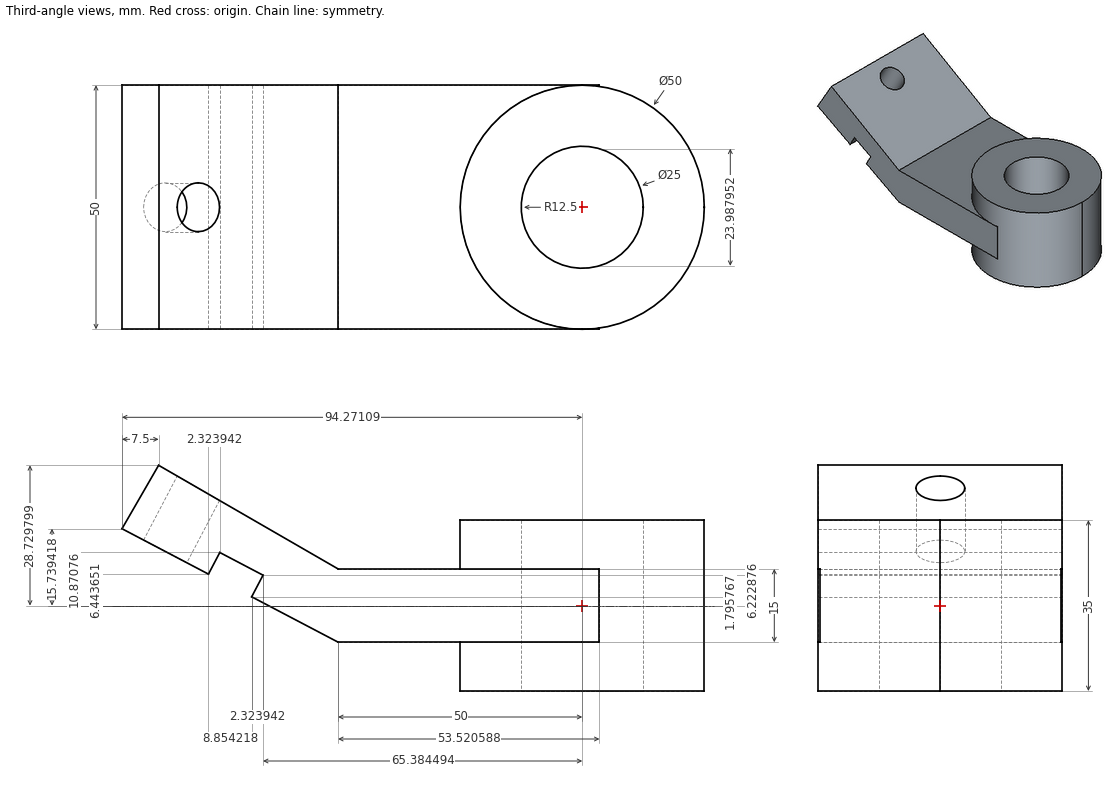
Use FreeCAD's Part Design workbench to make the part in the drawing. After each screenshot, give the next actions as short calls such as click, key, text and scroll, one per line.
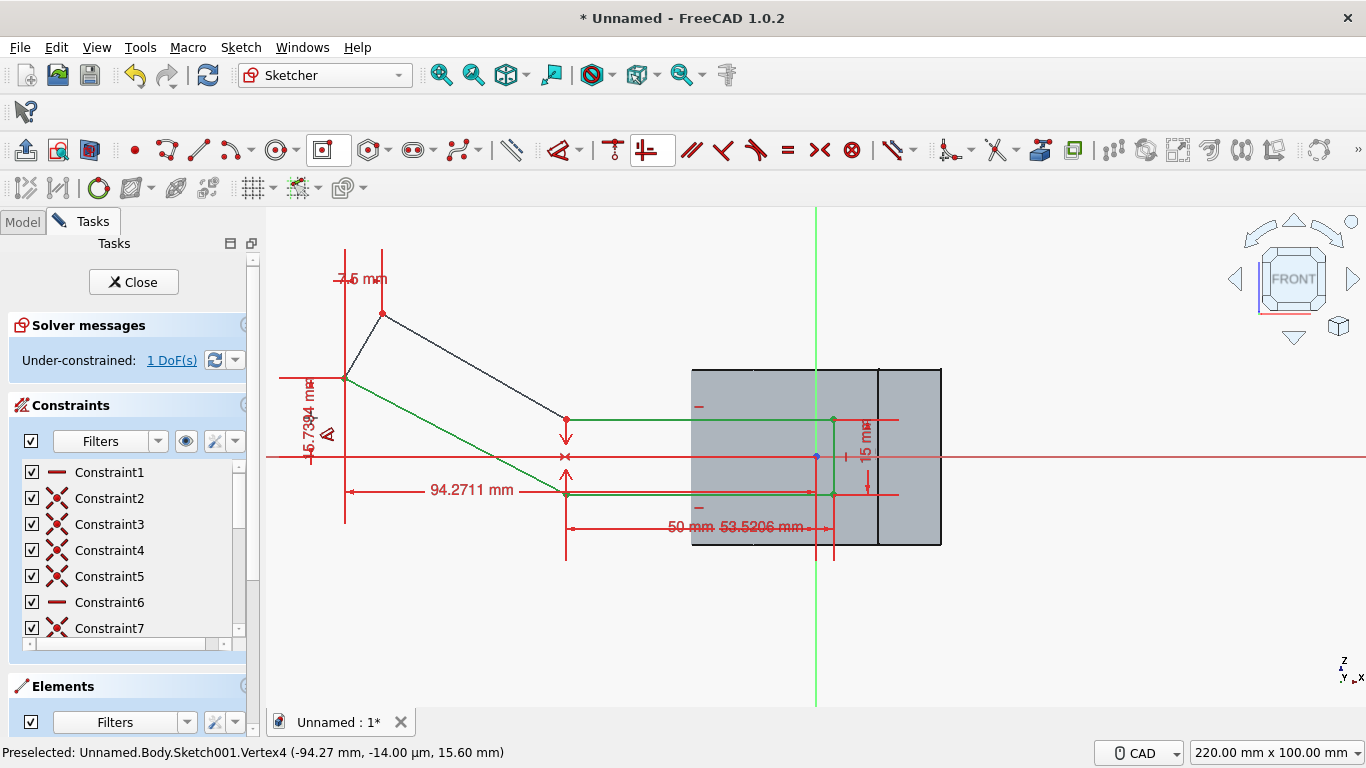
click(382, 314)
click(850, 385)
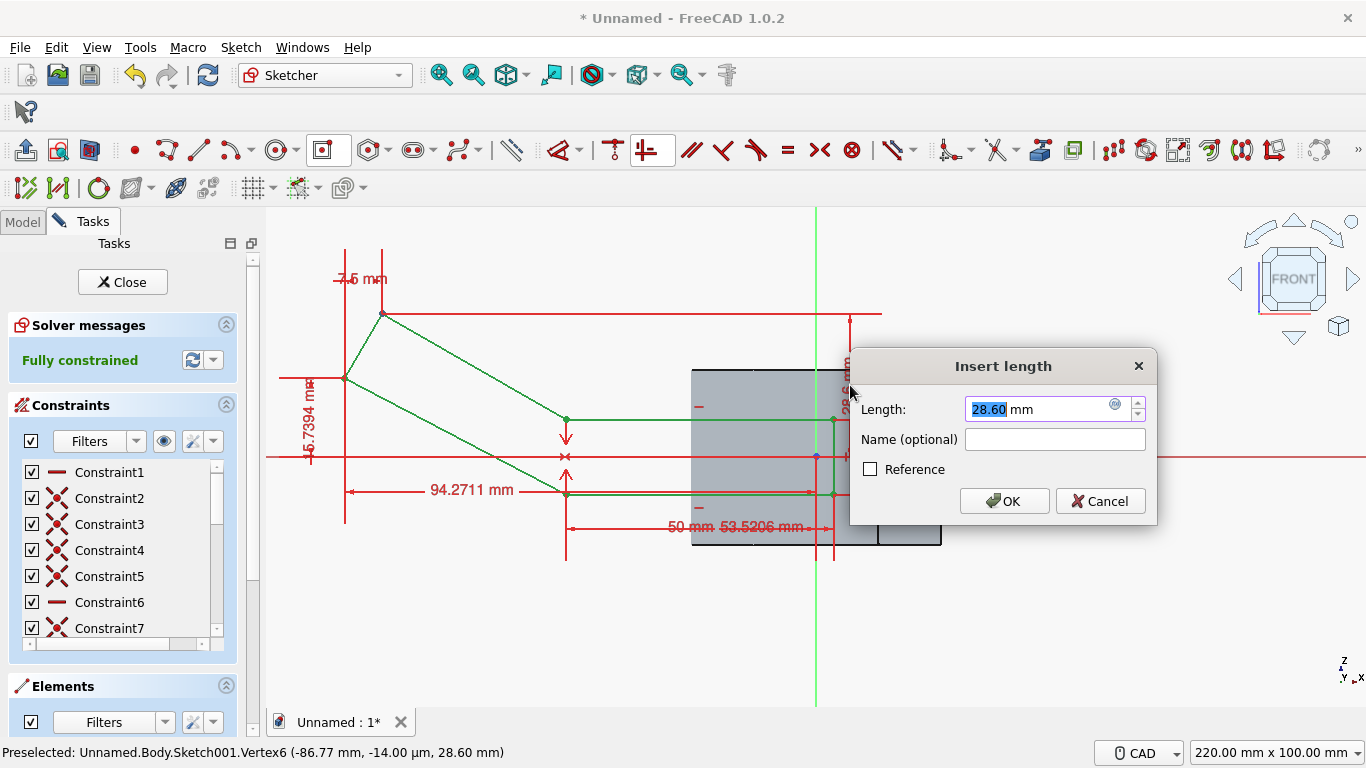
text(28.729799)
key(Return)
key(Escape)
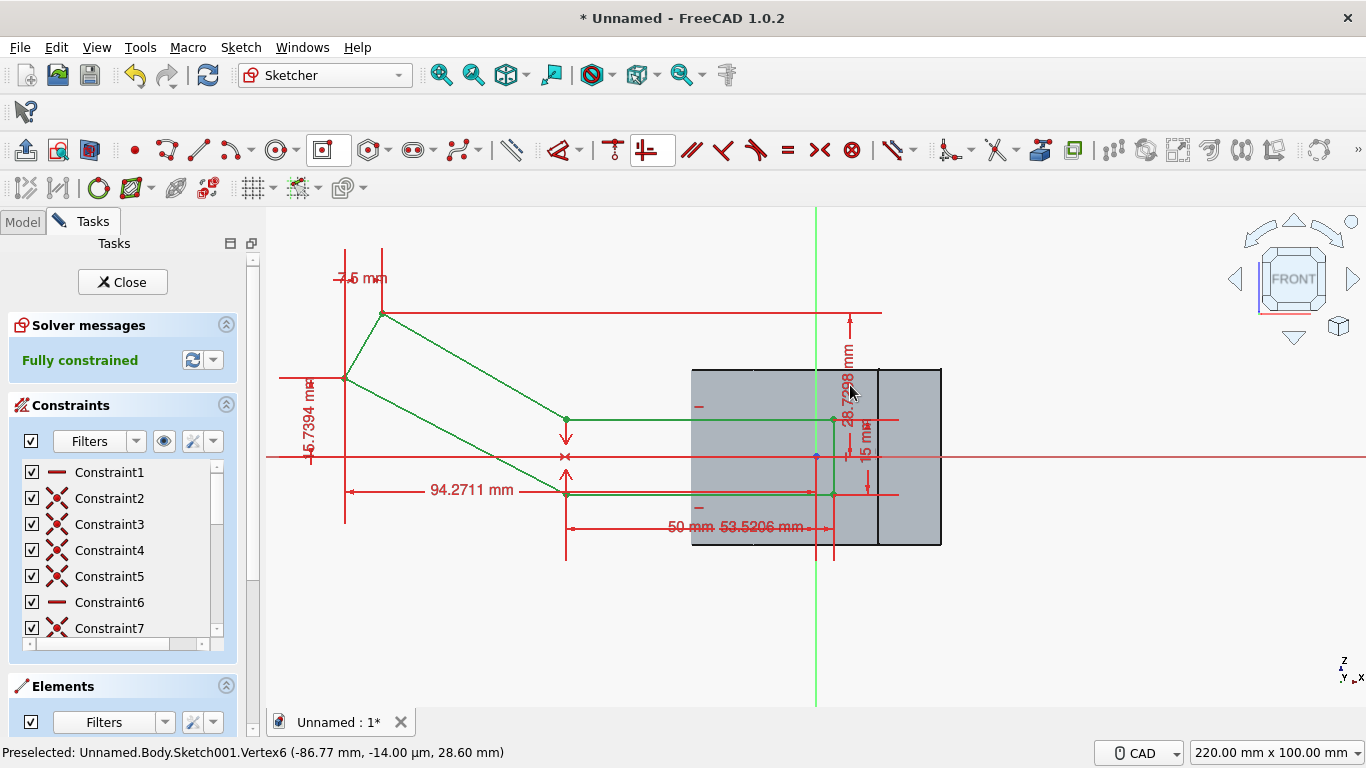
click(123, 282)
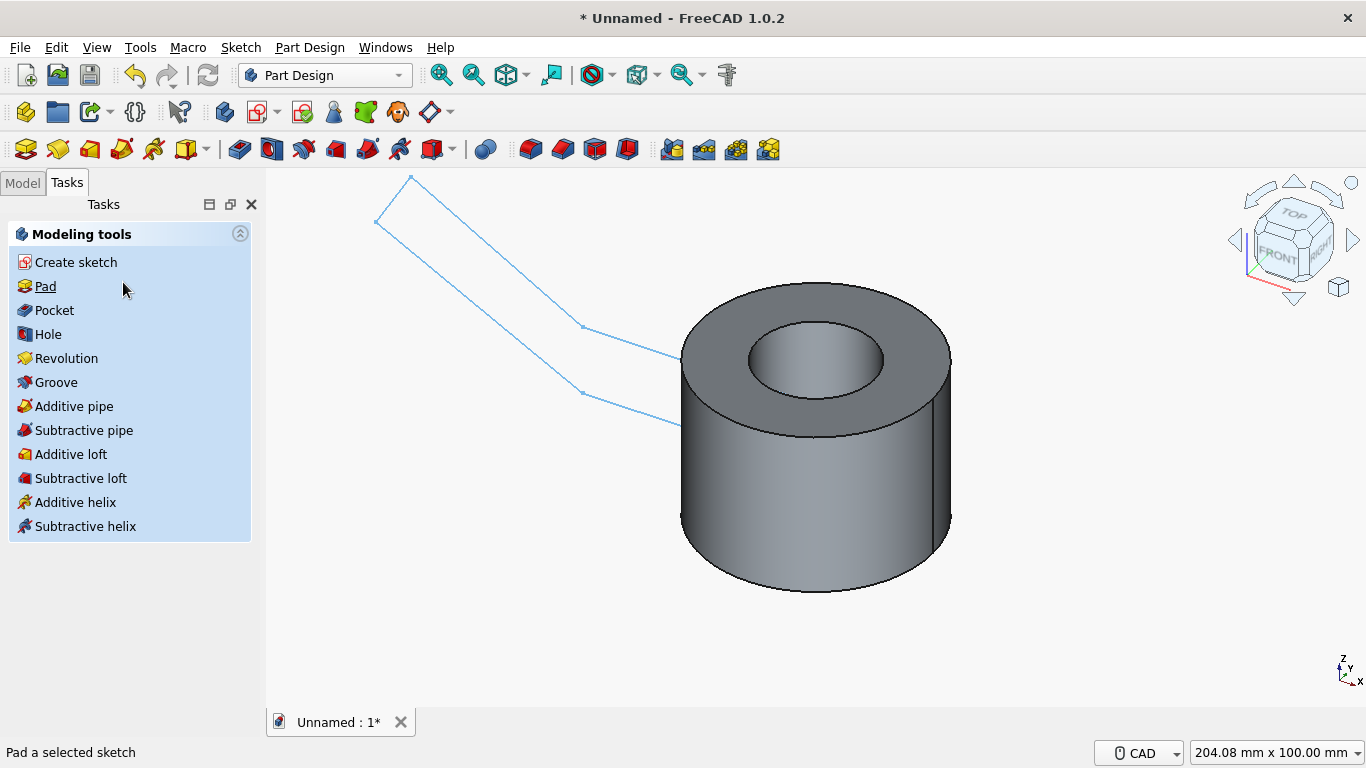
click(26, 150)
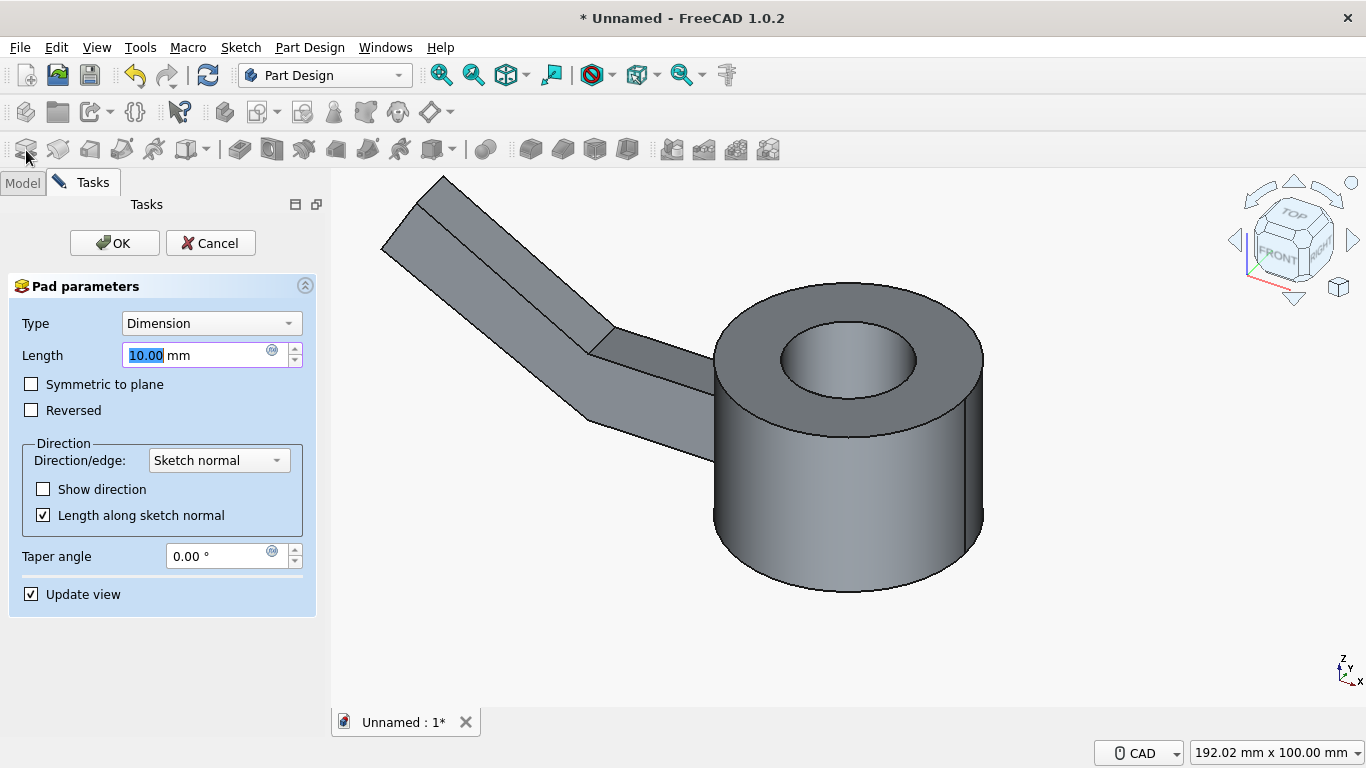
text(50)
key(Tab)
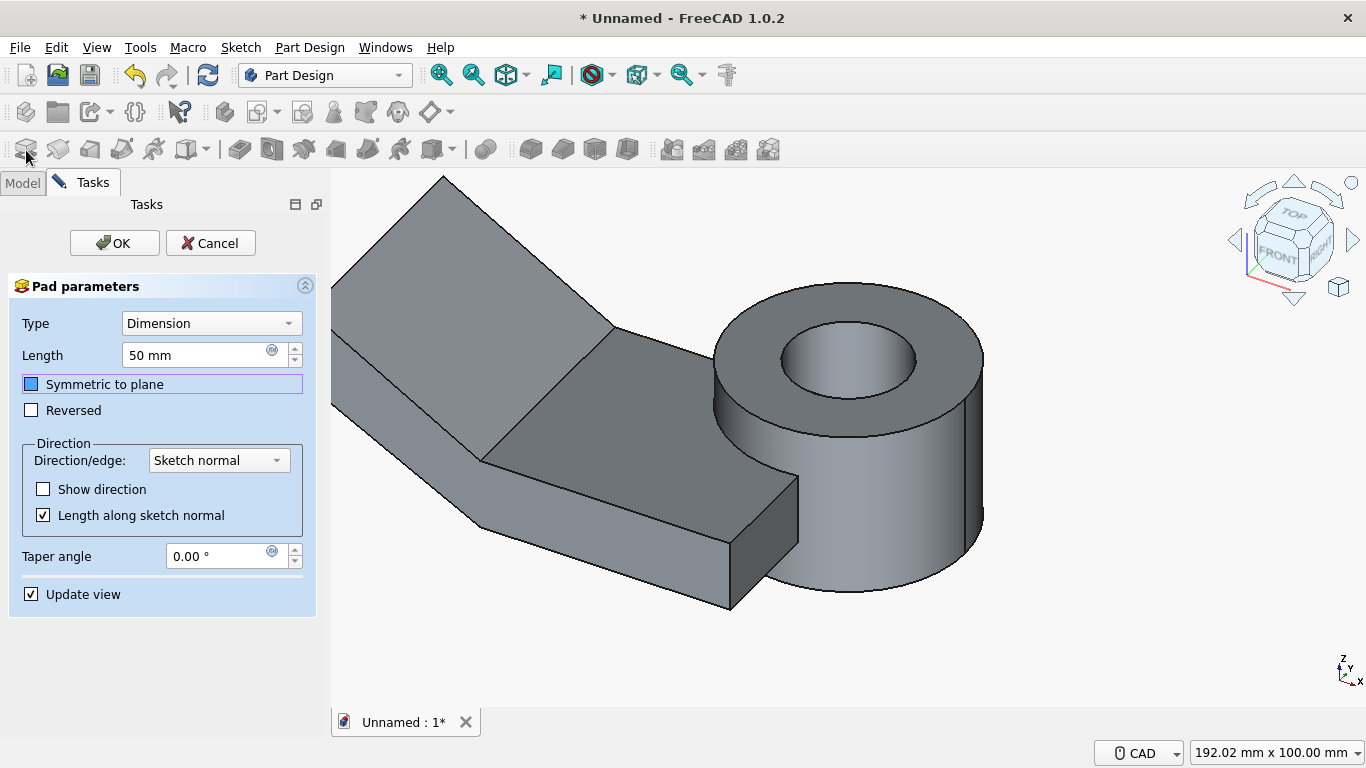
click(30, 384)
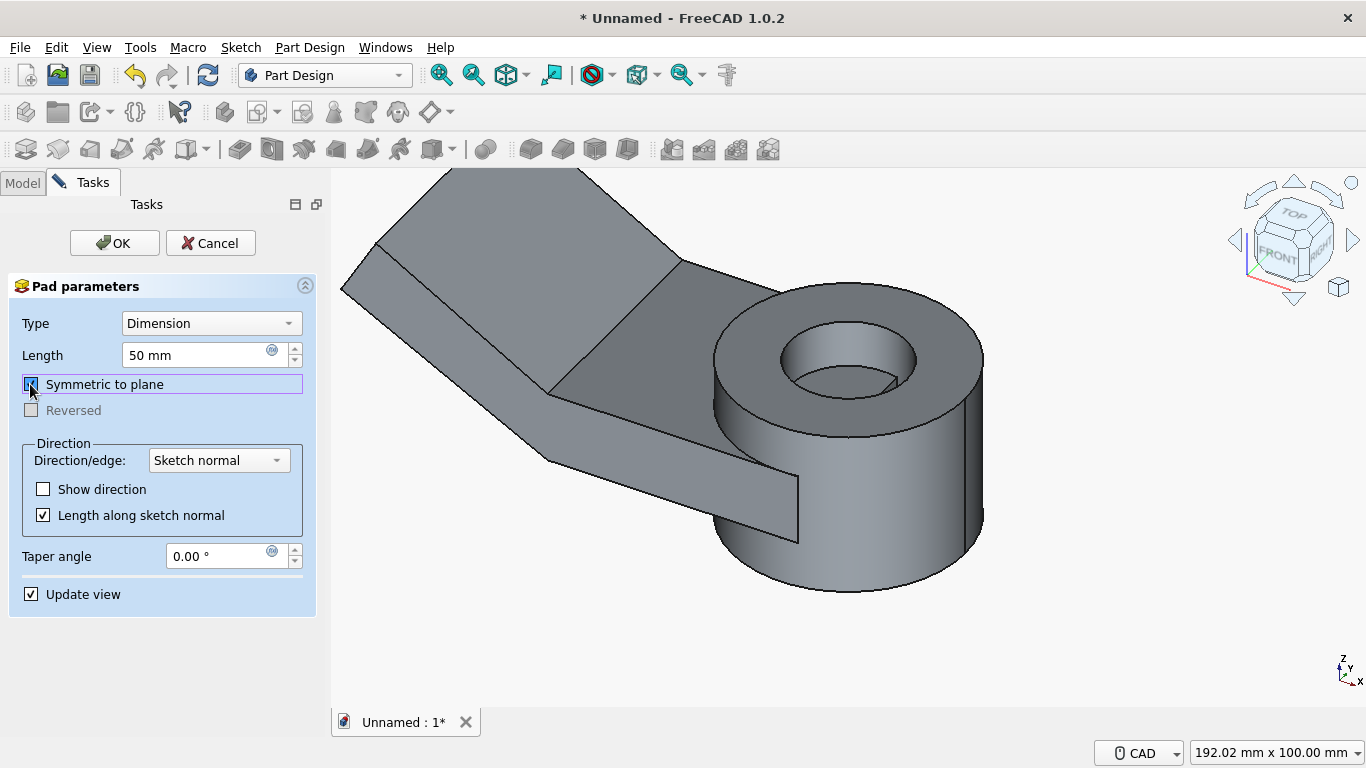
click(115, 243)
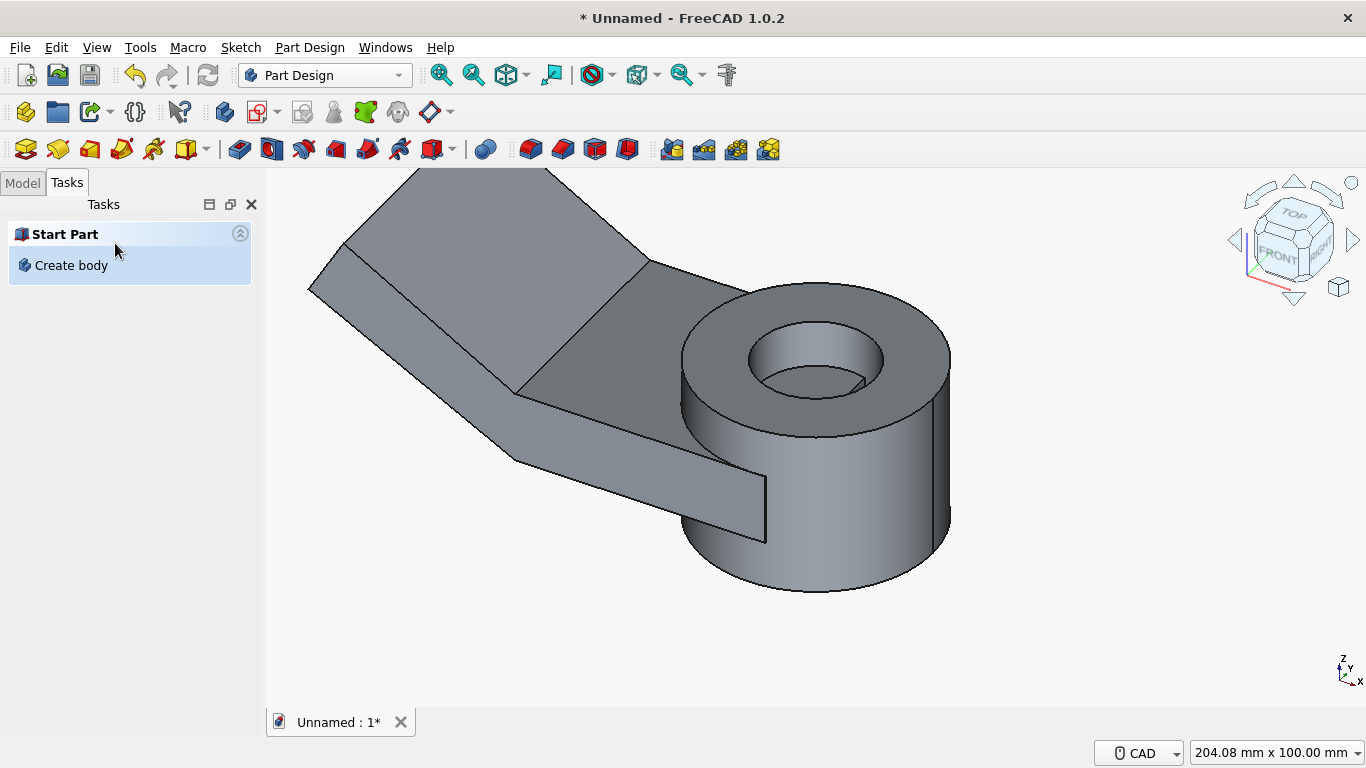
click(442, 76)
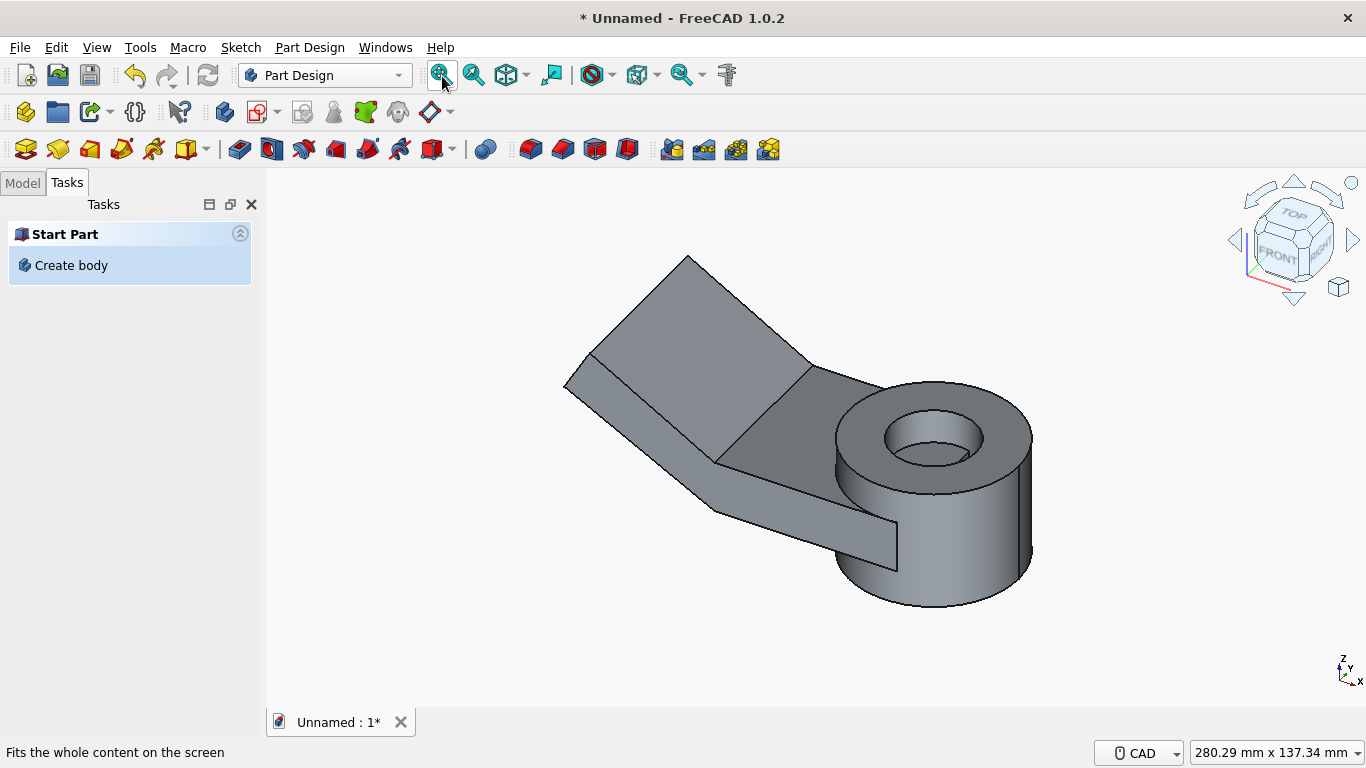
key(4)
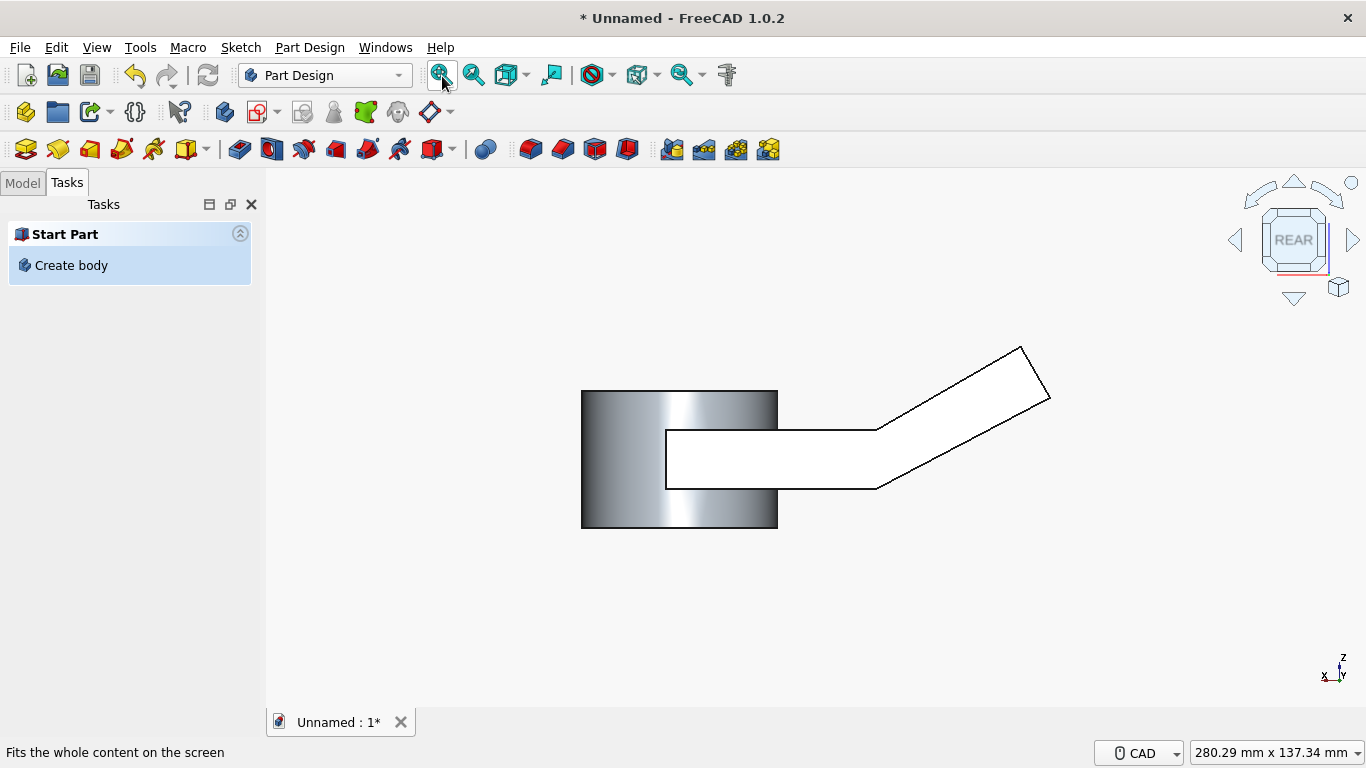
click(442, 76)